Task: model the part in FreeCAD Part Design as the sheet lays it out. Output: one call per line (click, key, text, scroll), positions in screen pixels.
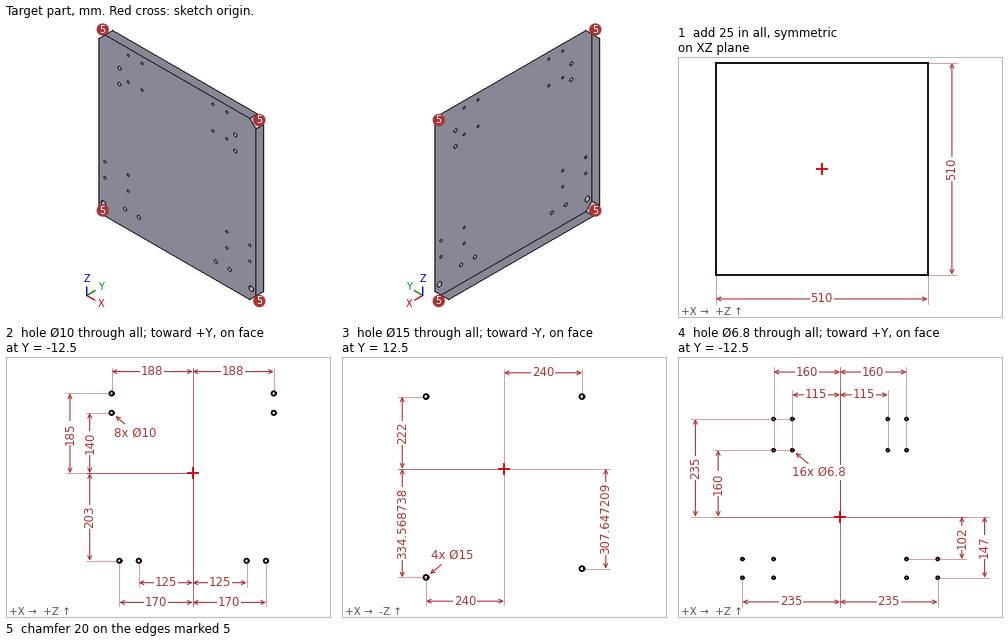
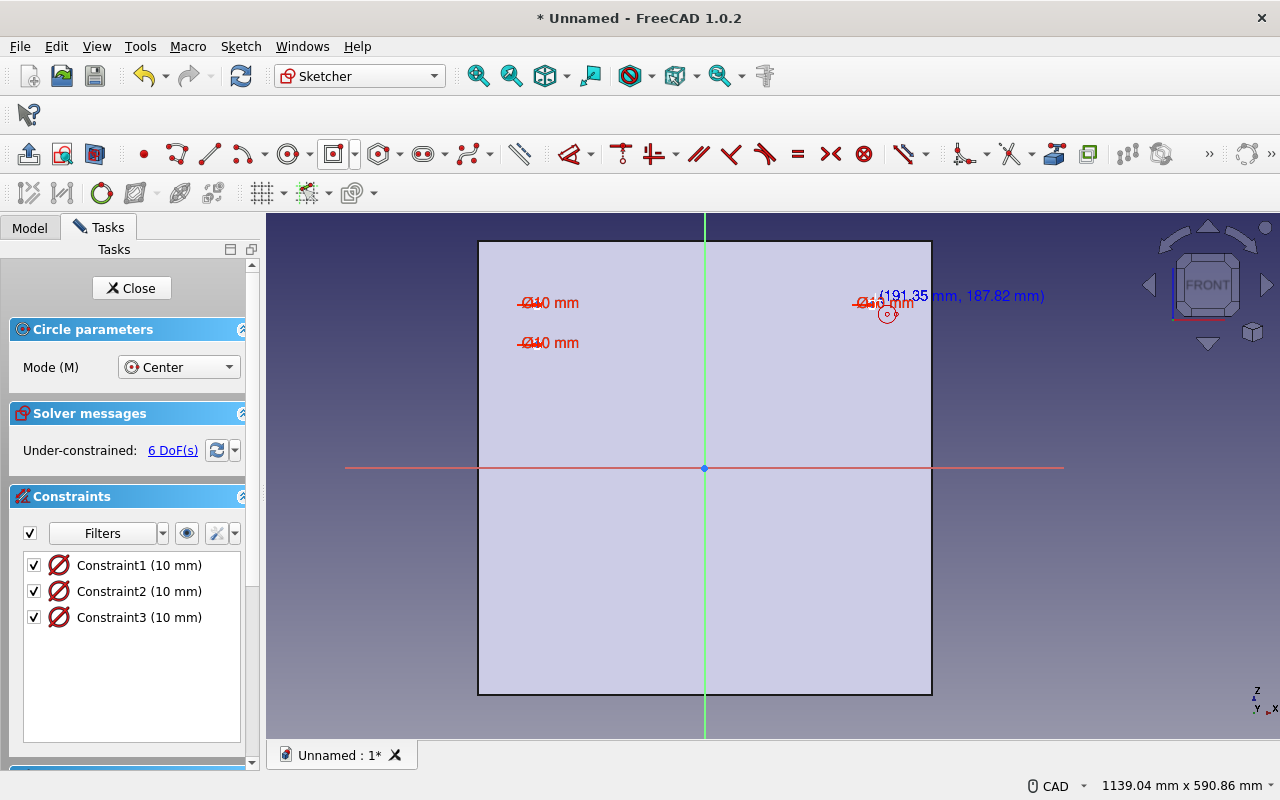
scroll(872, 344, up, 9)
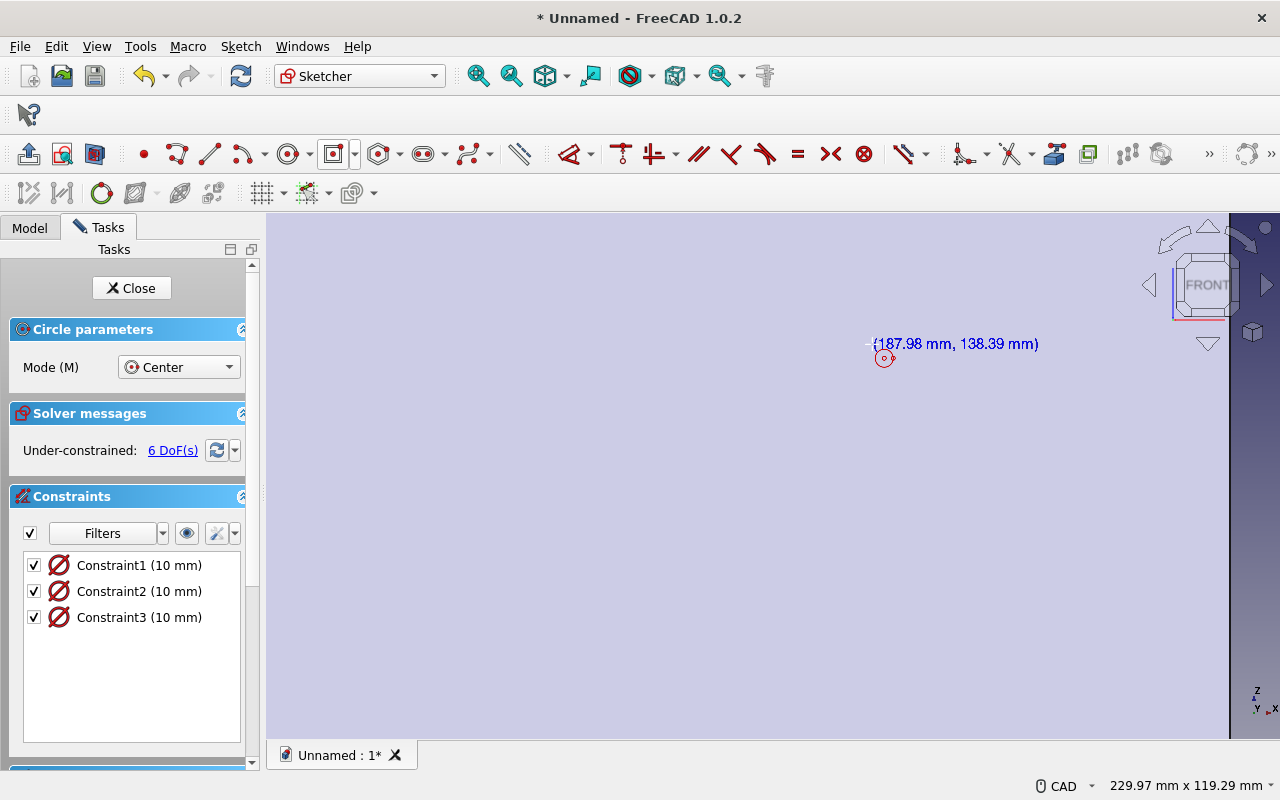
scroll(872, 344, down, 9)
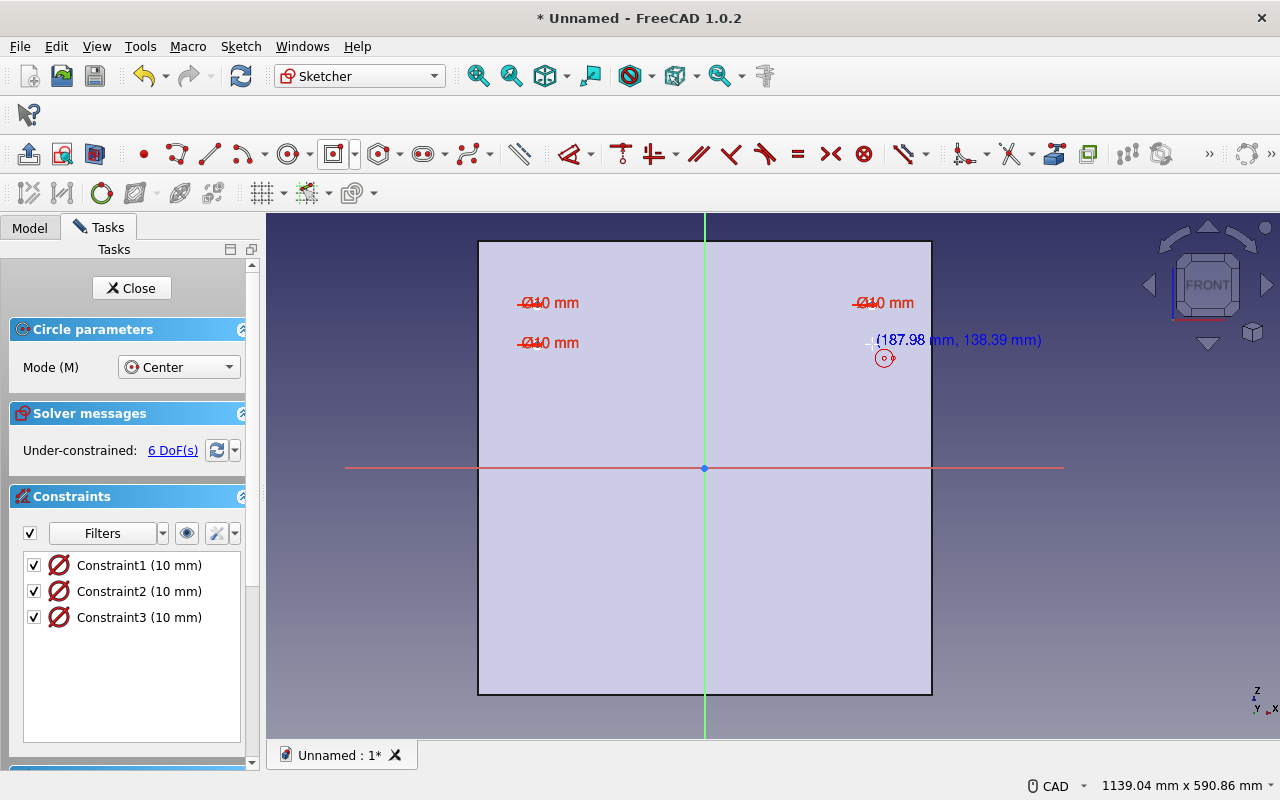
click(872, 344)
move(875, 340)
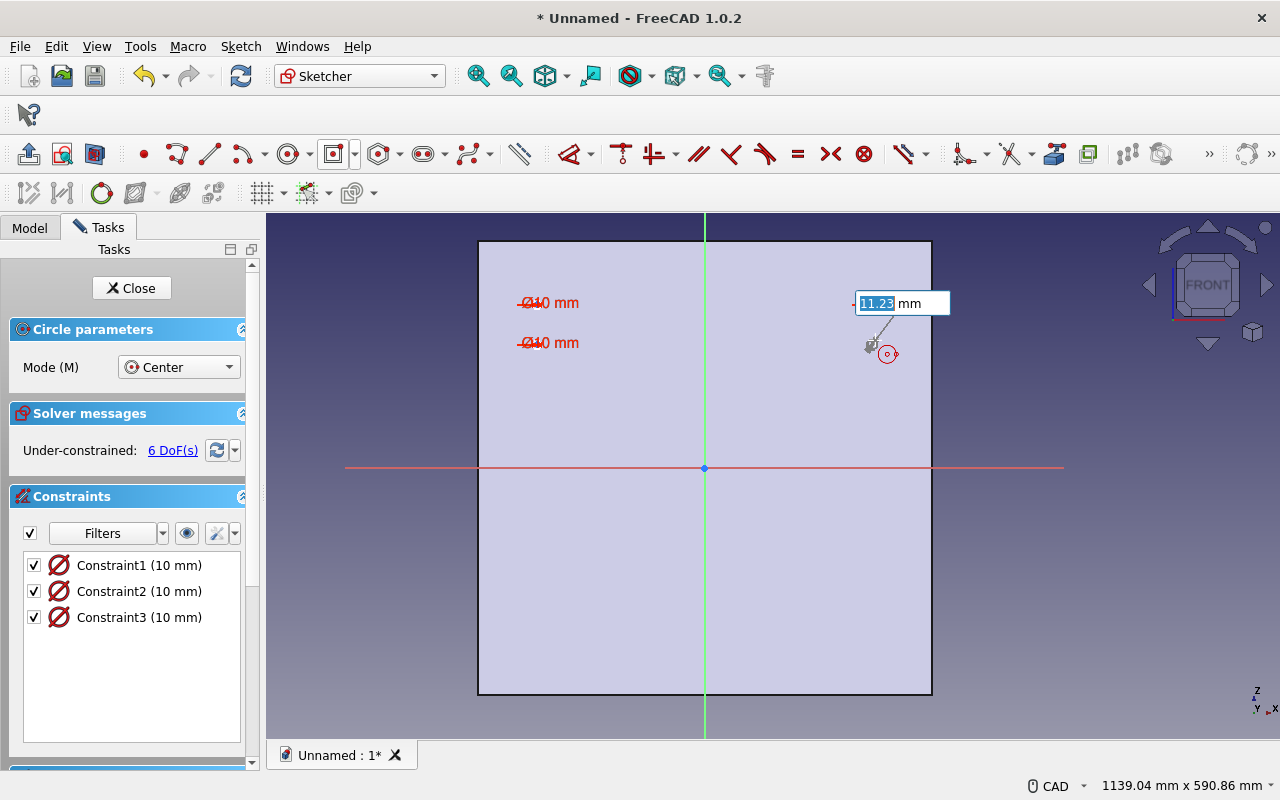
text(10)
key(Return)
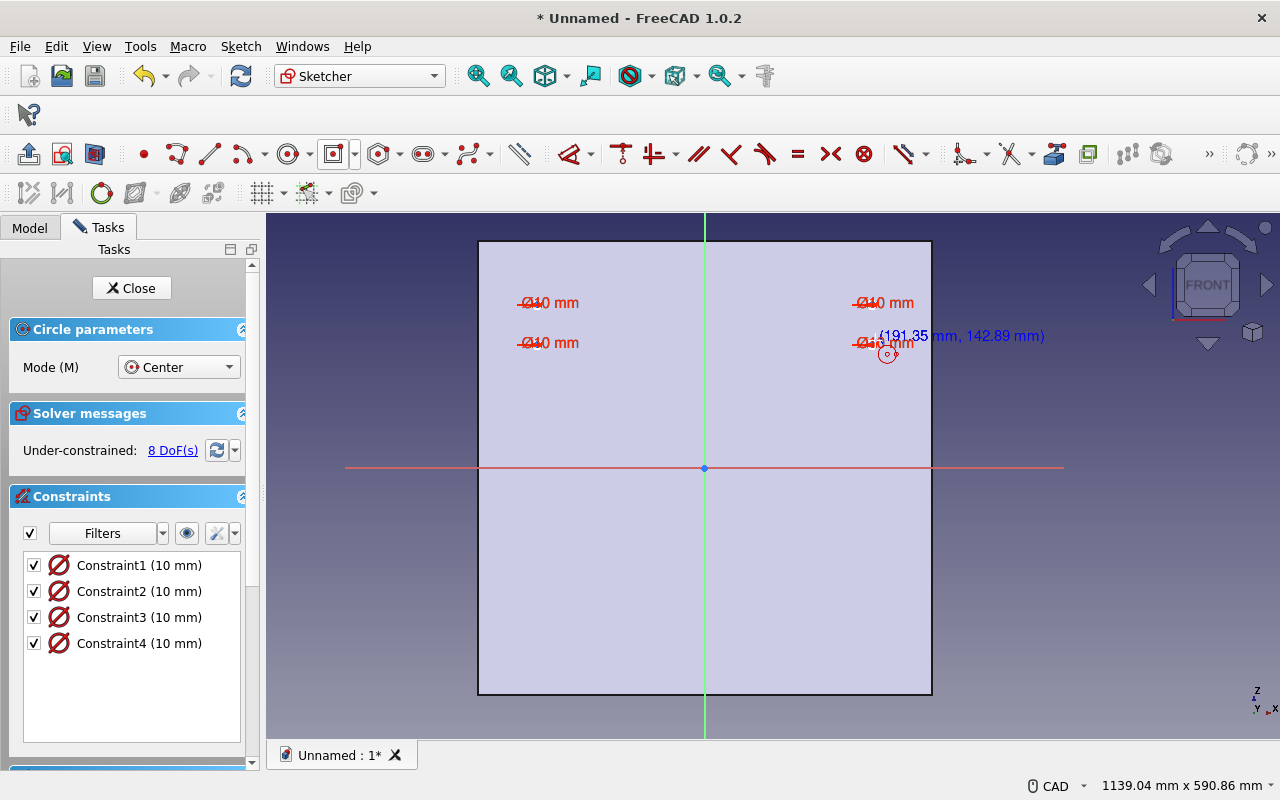
scroll(553, 649, up, 9)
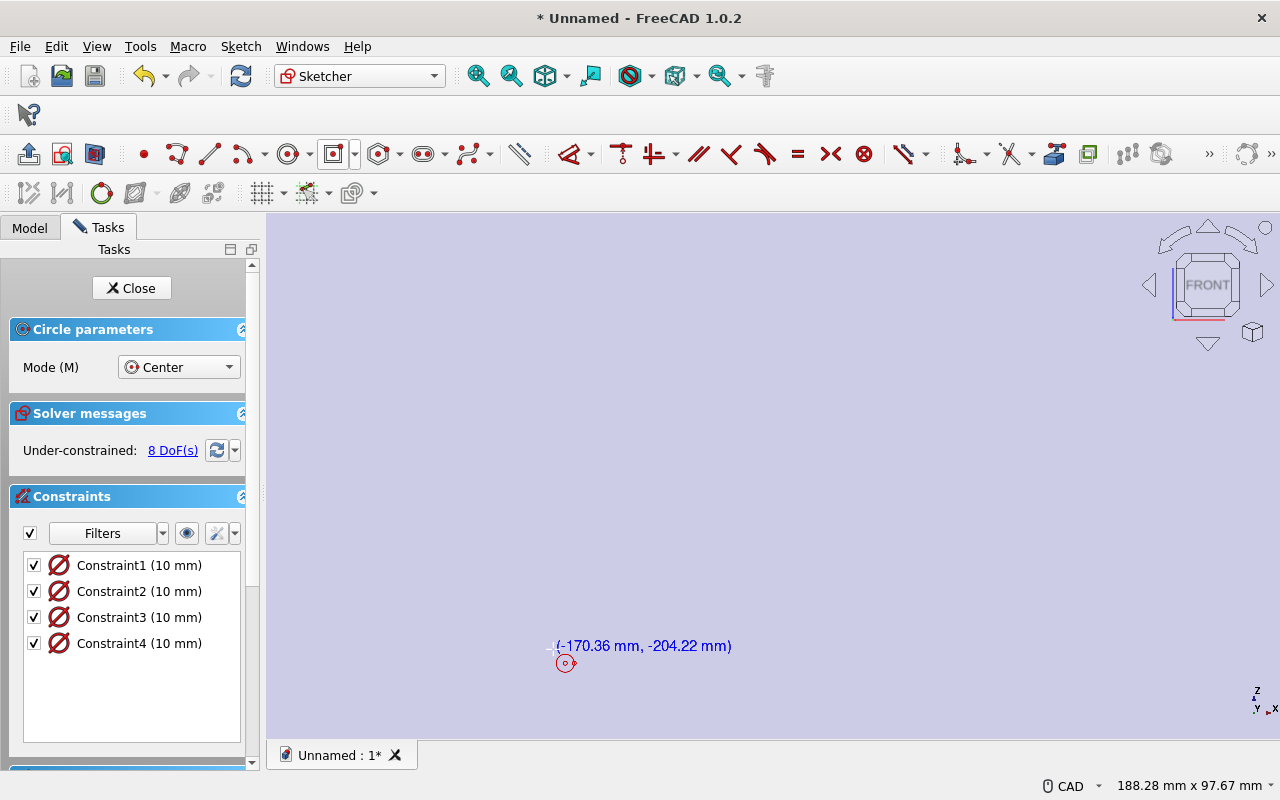
scroll(553, 650, down, 9)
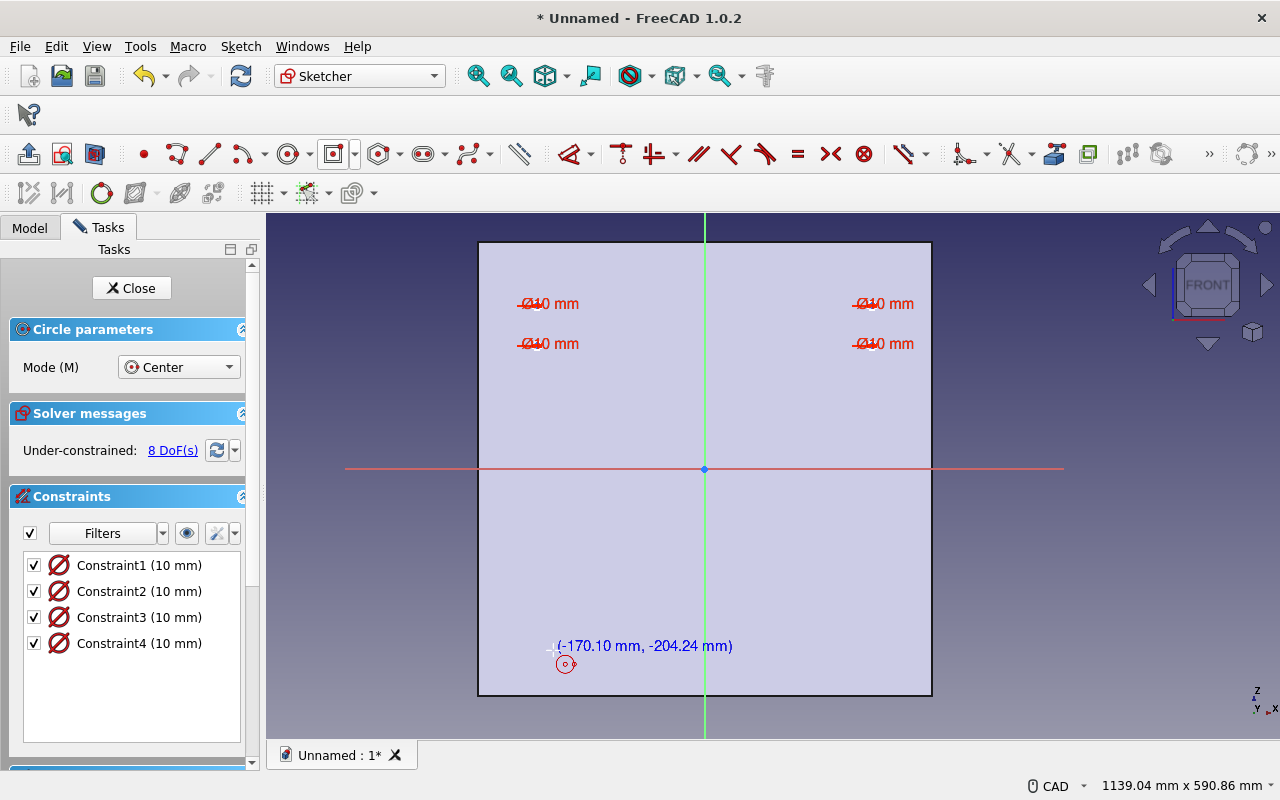
click(553, 650)
move(556, 647)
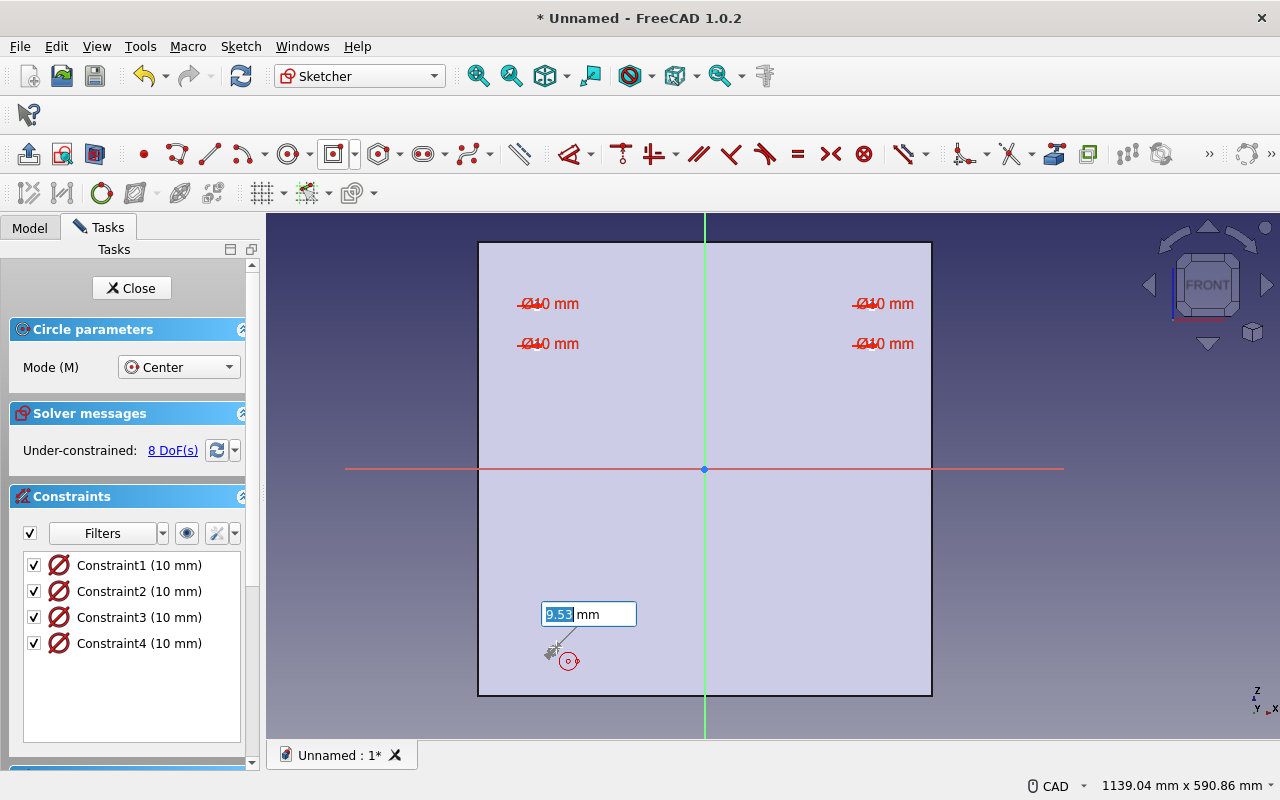
text(10)
key(Return)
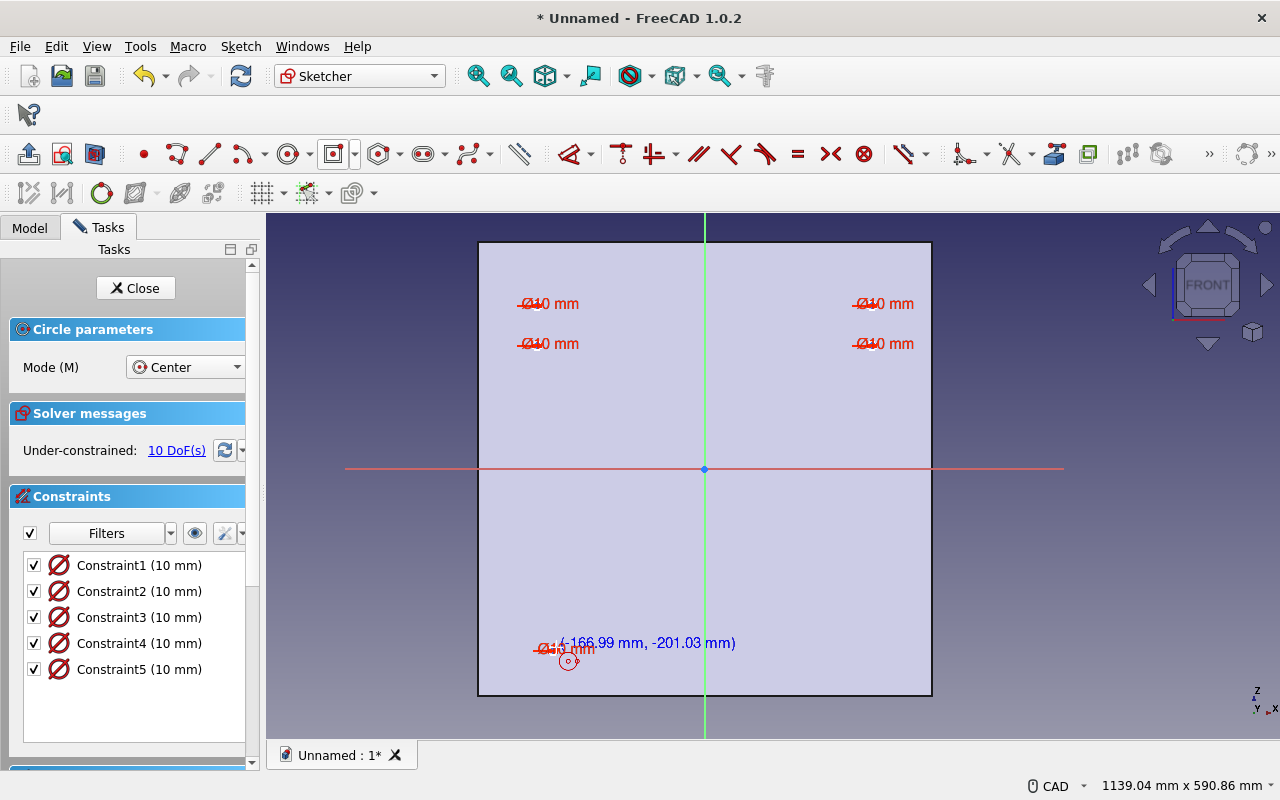
scroll(593, 650, up, 9)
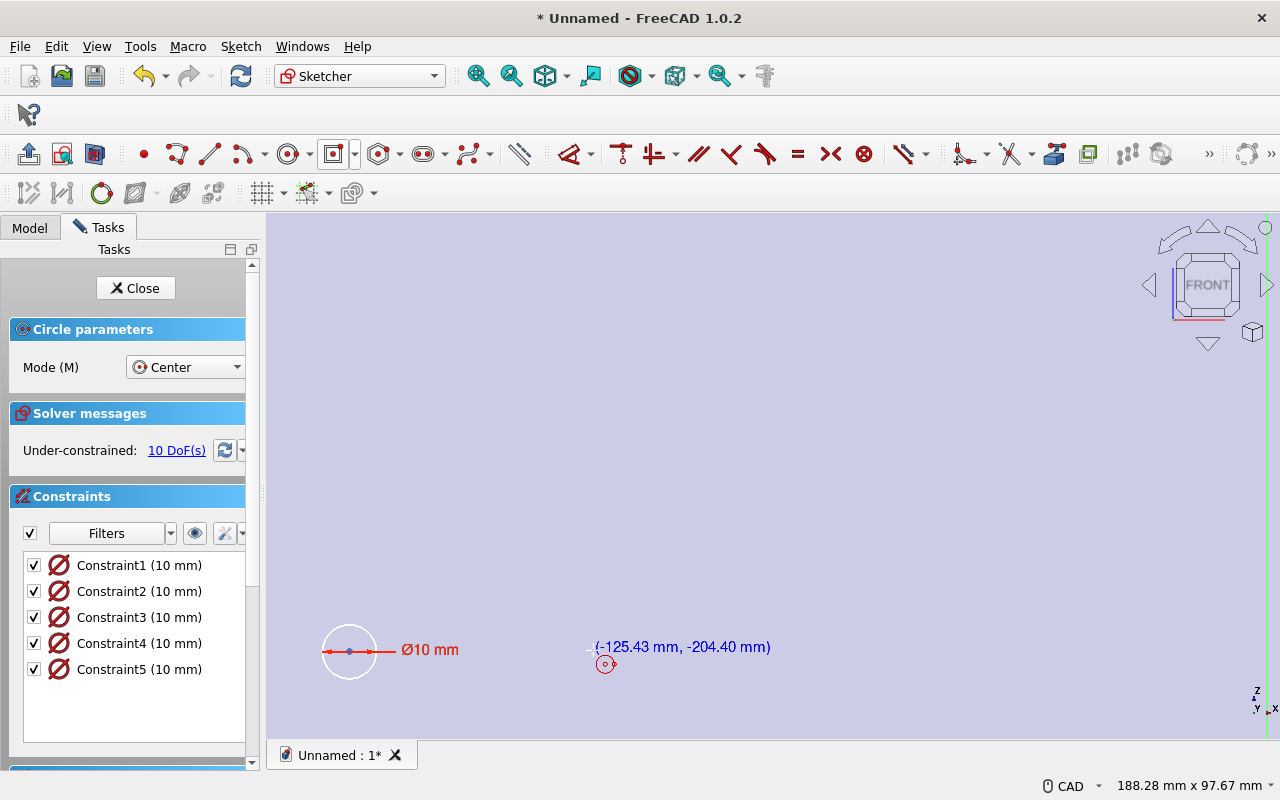
scroll(593, 650, down, 9)